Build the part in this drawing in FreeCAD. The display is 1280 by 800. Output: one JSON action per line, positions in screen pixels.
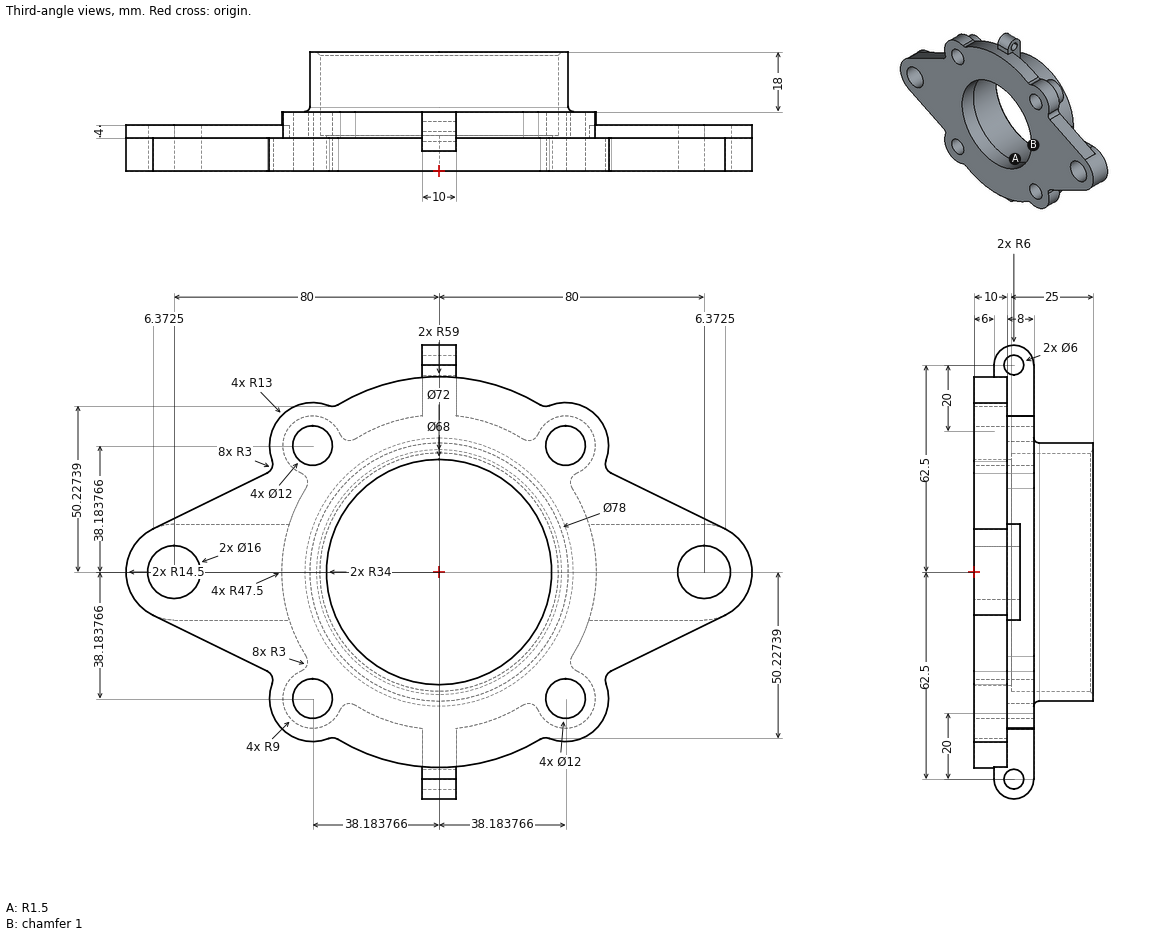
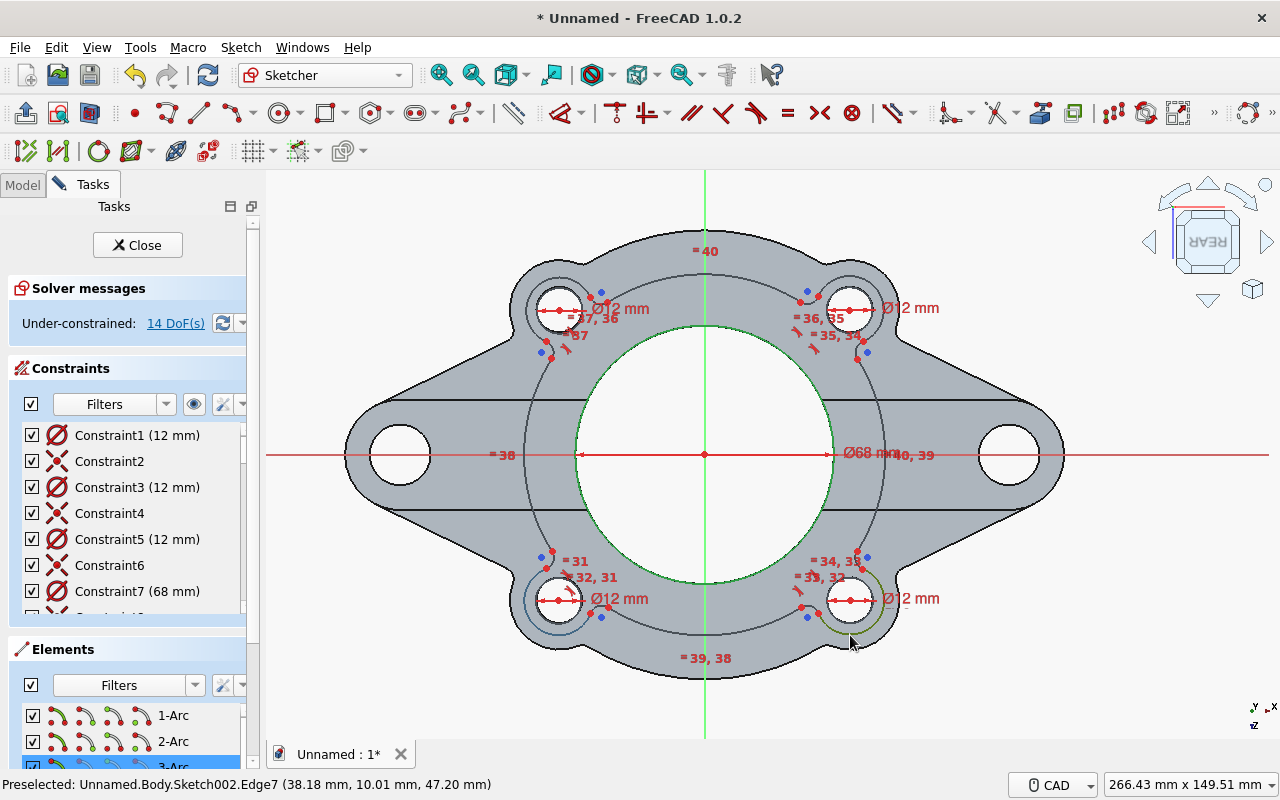
{"action": "left_click", "coordinate": [850, 276]}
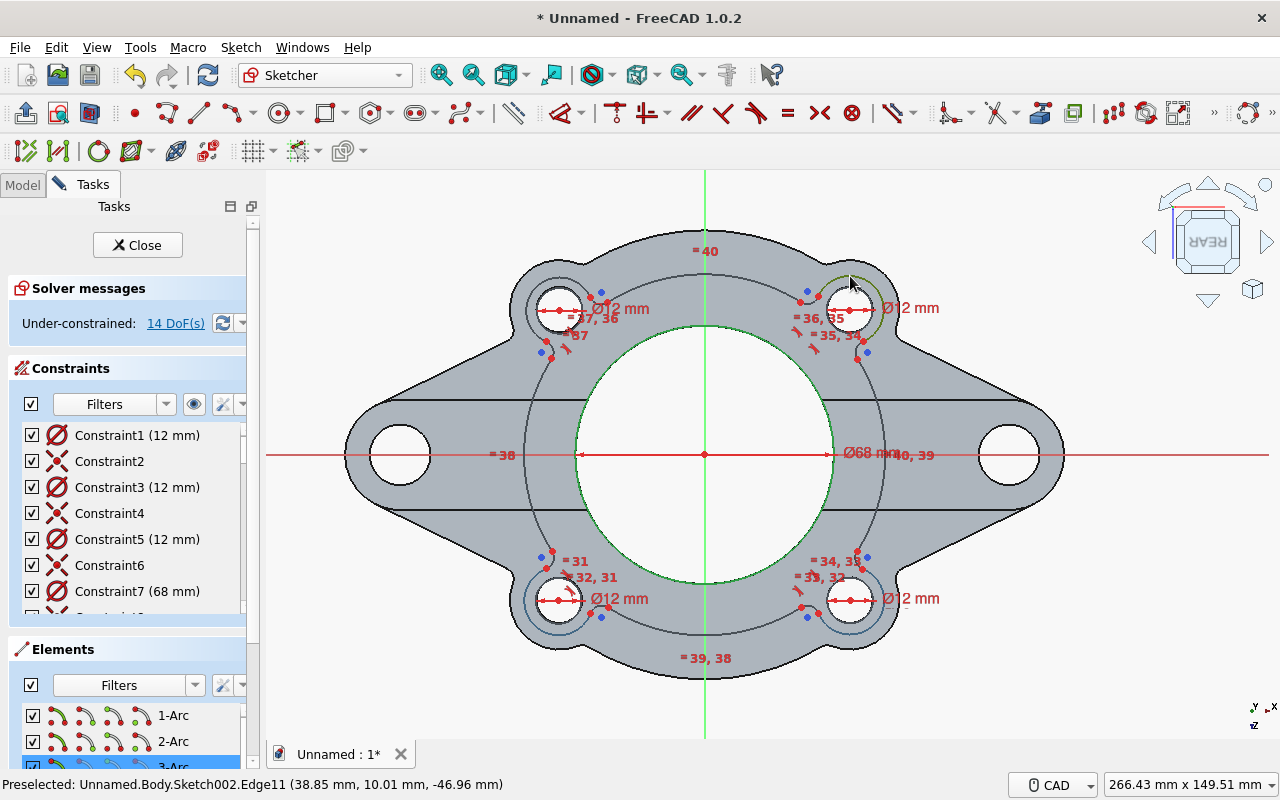
{"action": "scroll", "coordinate": [559, 277], "scroll_direction": "up", "scroll_amount": 2}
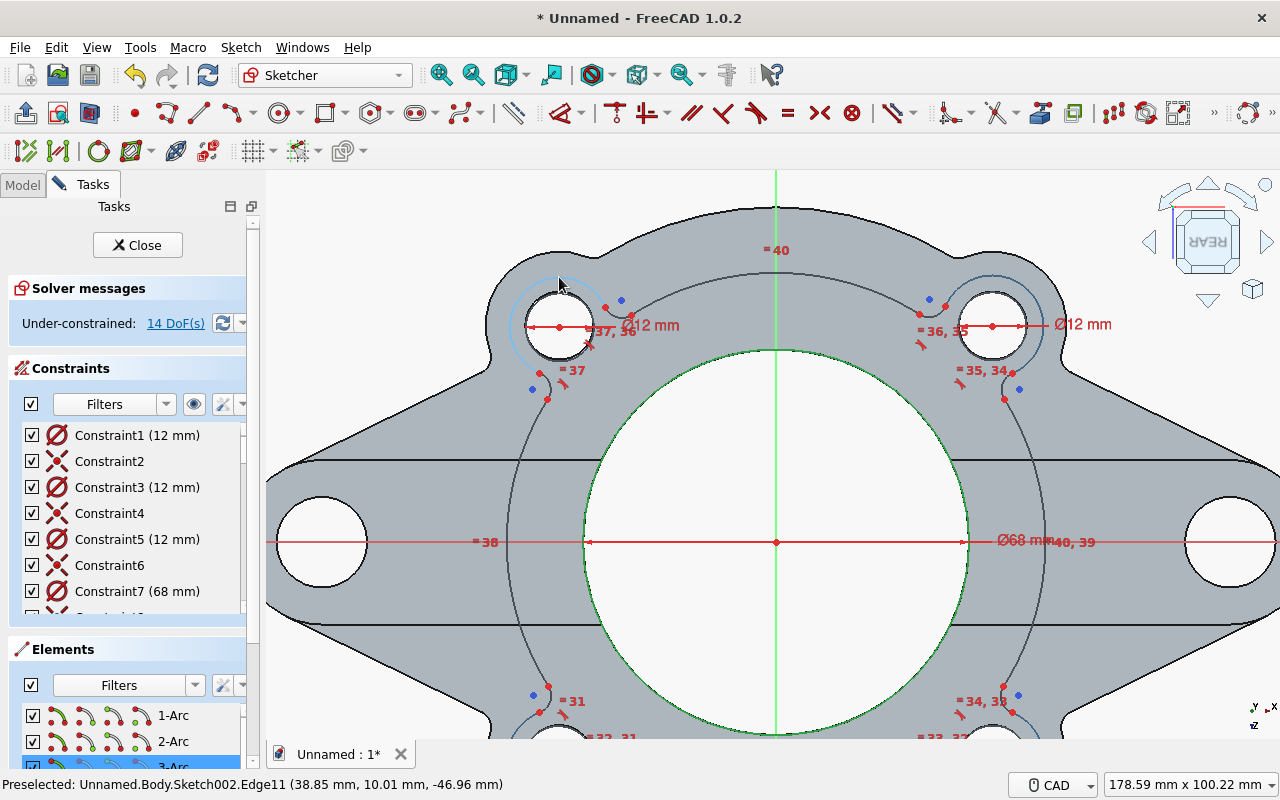
{"action": "left_click", "coordinate": [559, 278]}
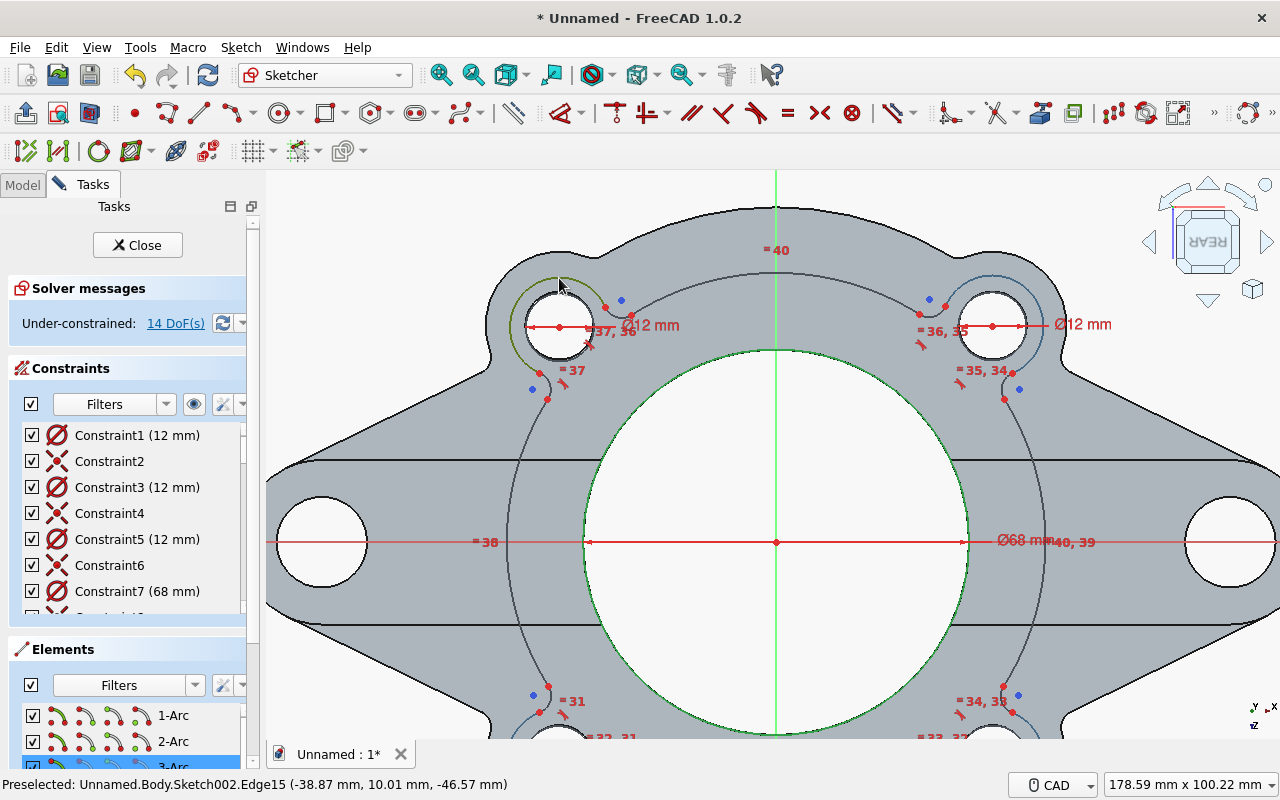
{"action": "left_click", "coordinate": [788, 114]}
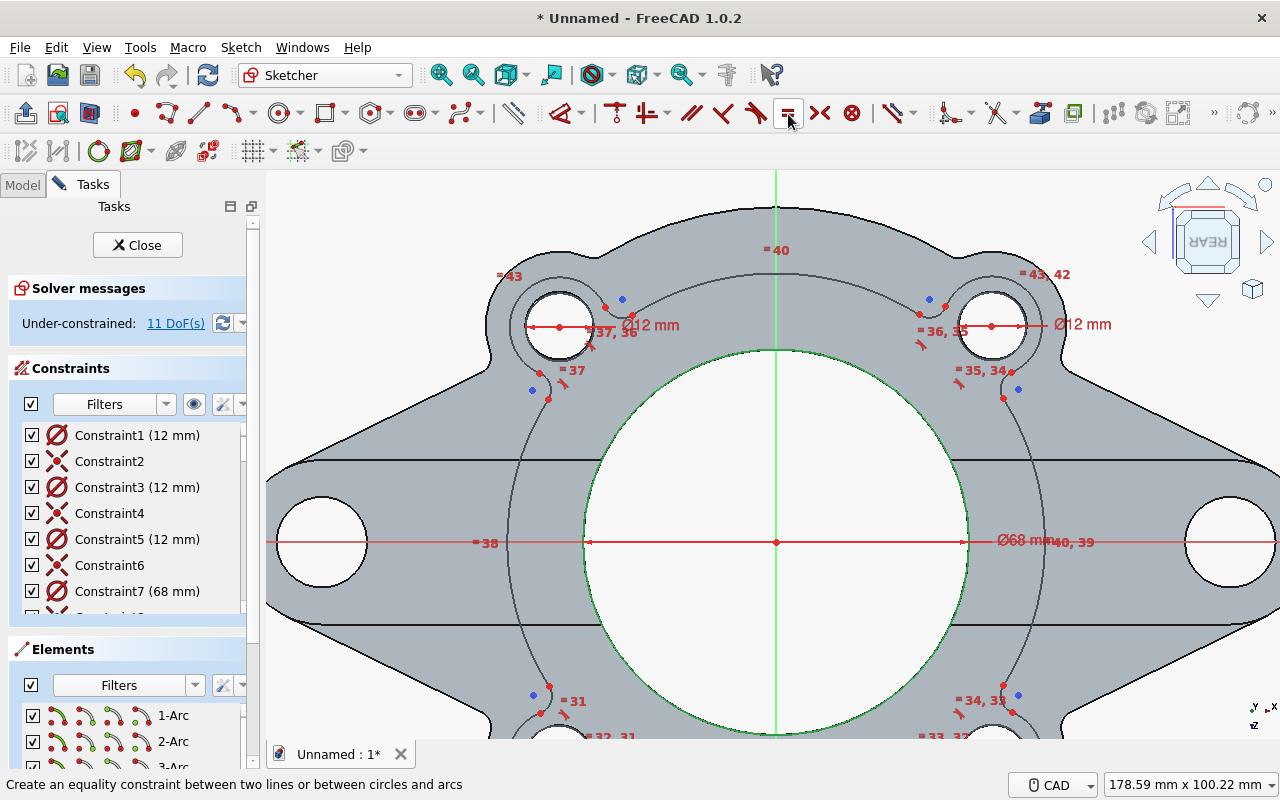
{"action": "left_click", "coordinate": [560, 114]}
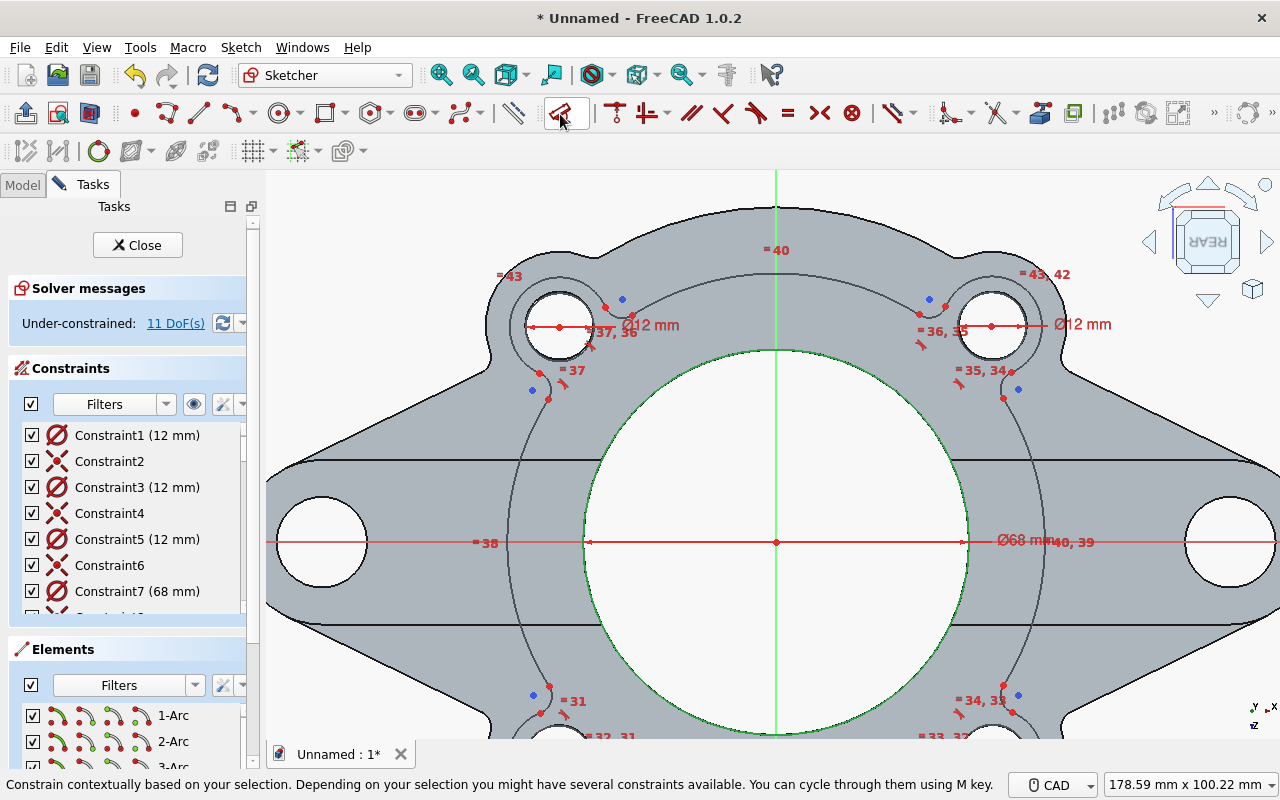
{"action": "left_click", "coordinate": [514, 483]}
{"action": "left_click", "coordinate": [483, 476]}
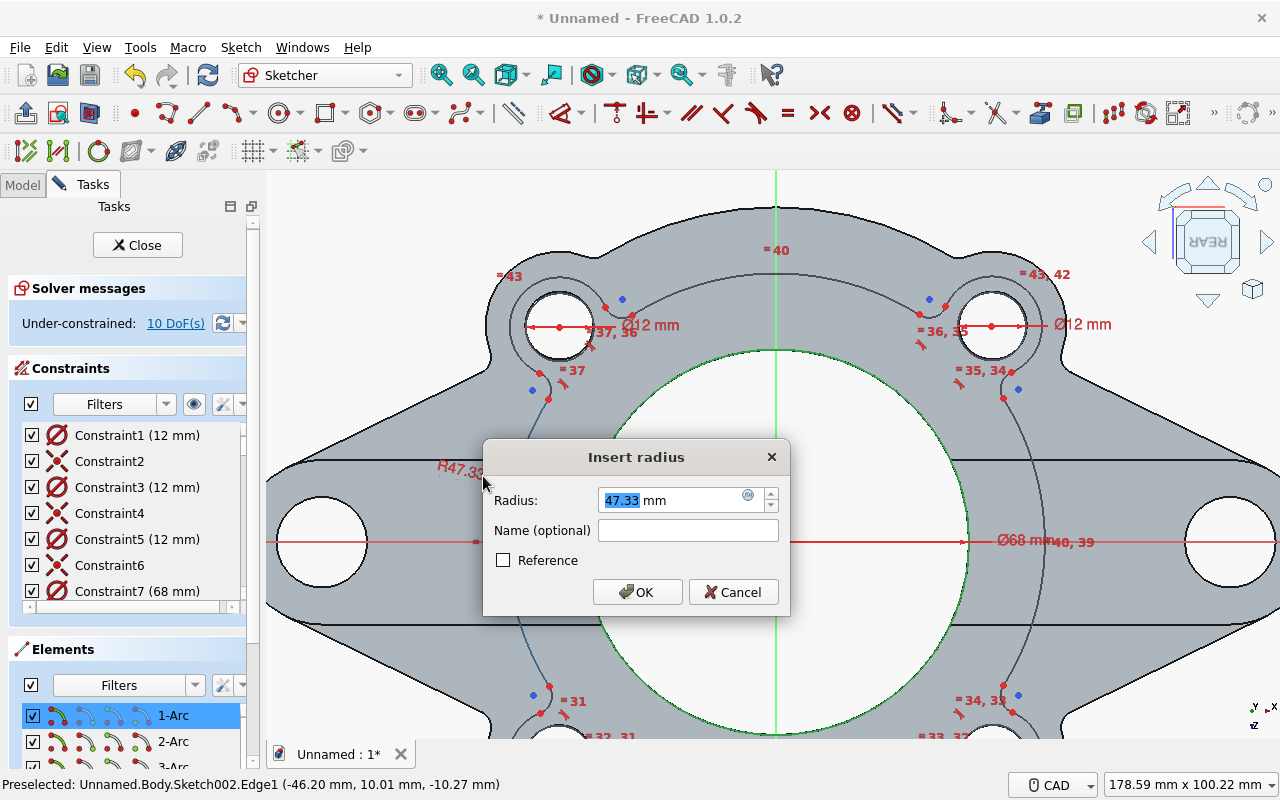
{"action": "type", "text": "47.5"}
{"action": "key", "text": "Return"}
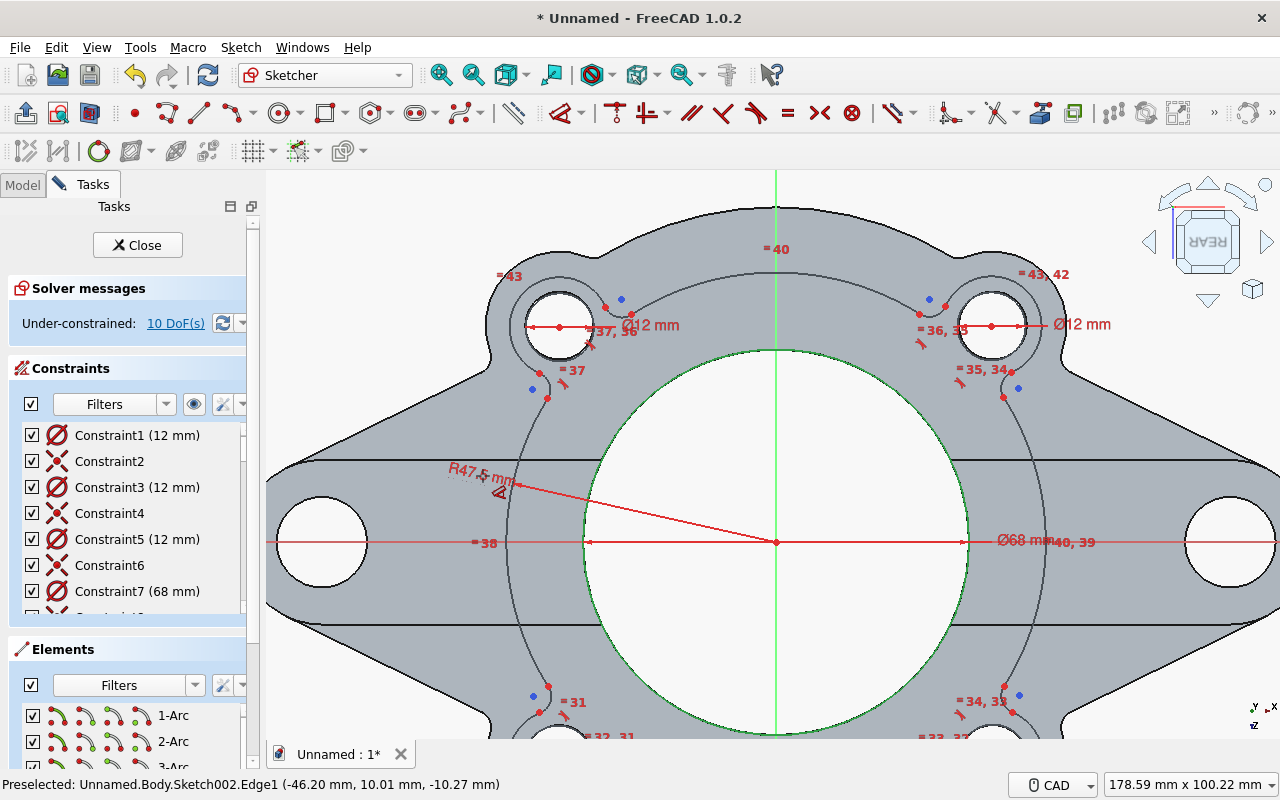
{"action": "scroll", "coordinate": [547, 707], "scroll_direction": "up", "scroll_amount": 5}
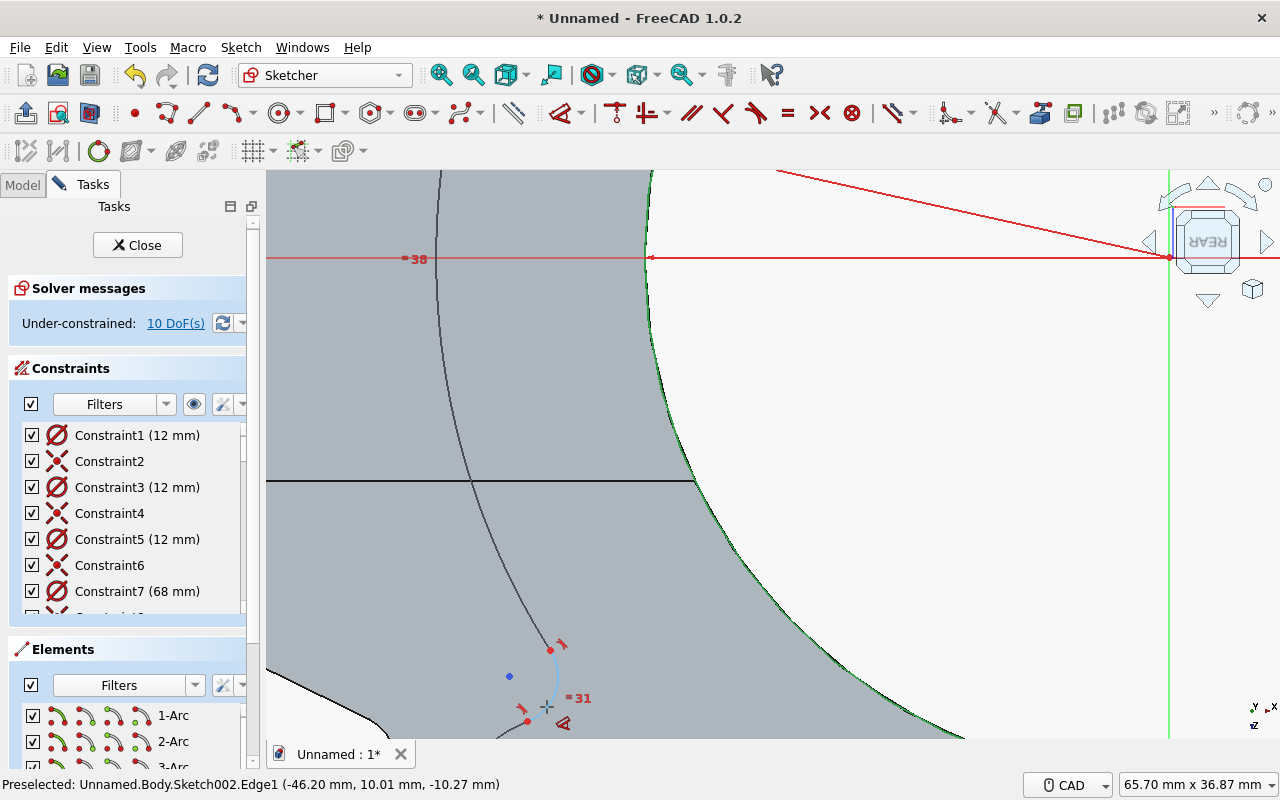
{"action": "left_click", "coordinate": [548, 707]}
{"action": "left_click", "coordinate": [589, 690]}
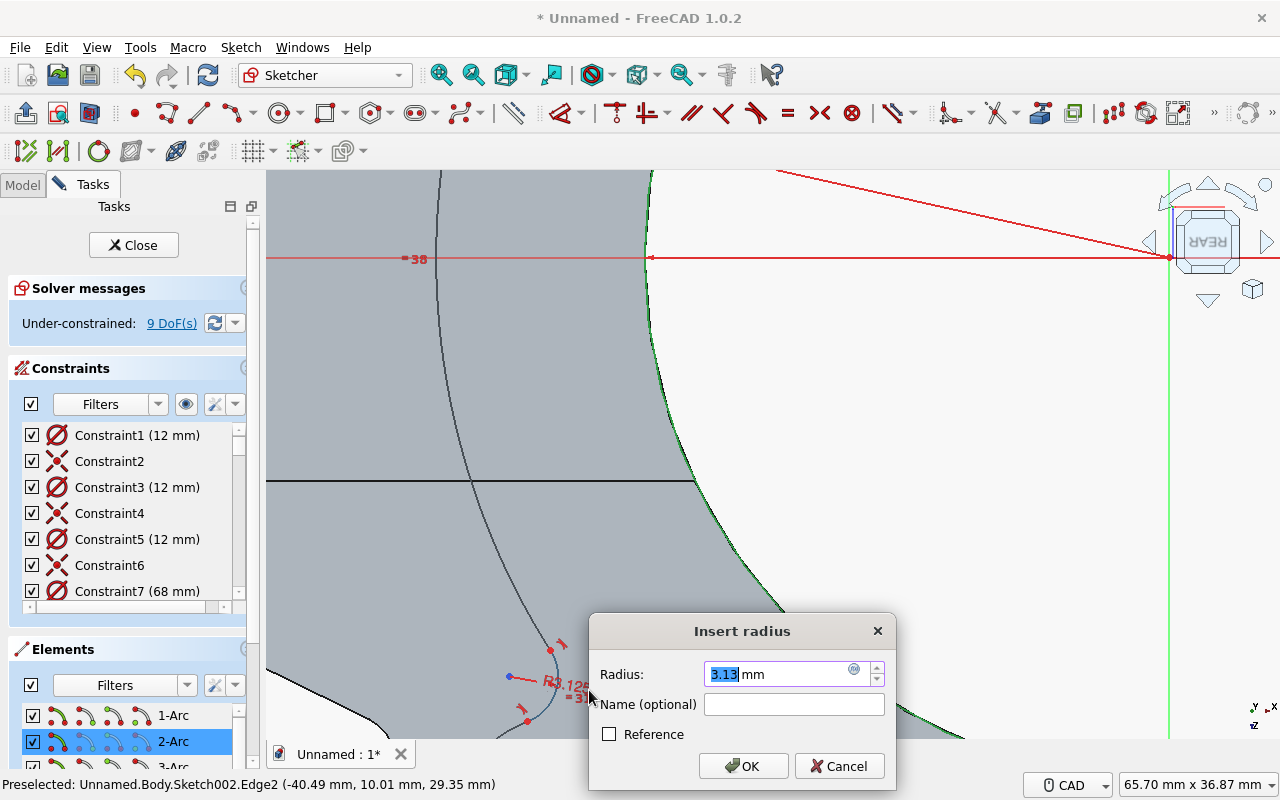
{"action": "type", "text": "3"}
{"action": "key", "text": "Return"}